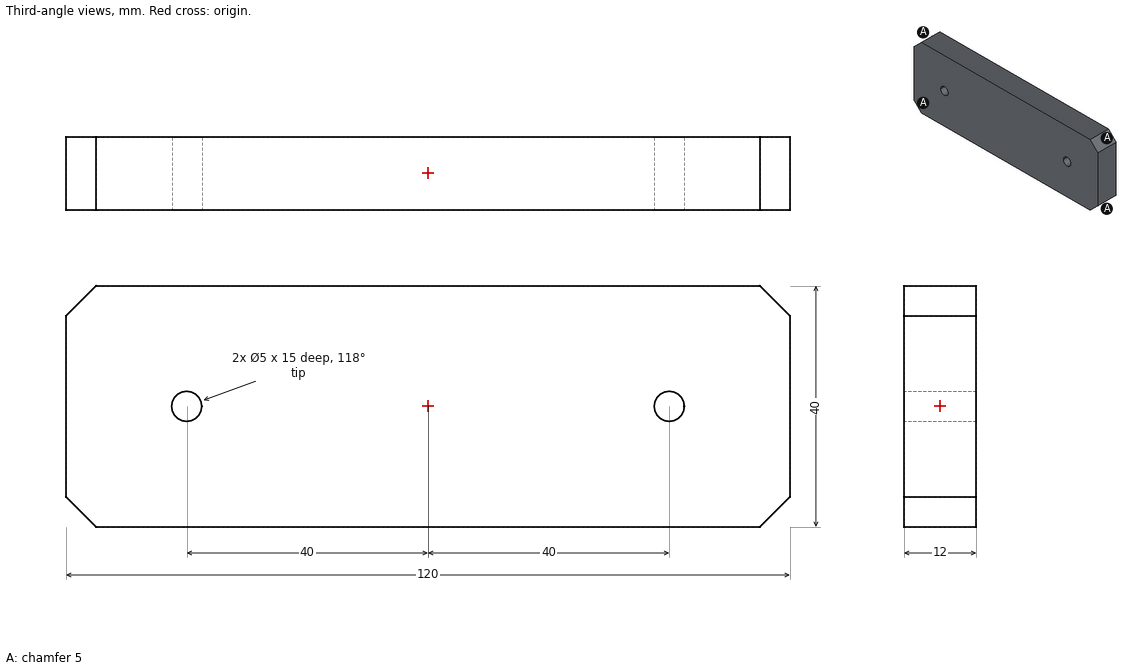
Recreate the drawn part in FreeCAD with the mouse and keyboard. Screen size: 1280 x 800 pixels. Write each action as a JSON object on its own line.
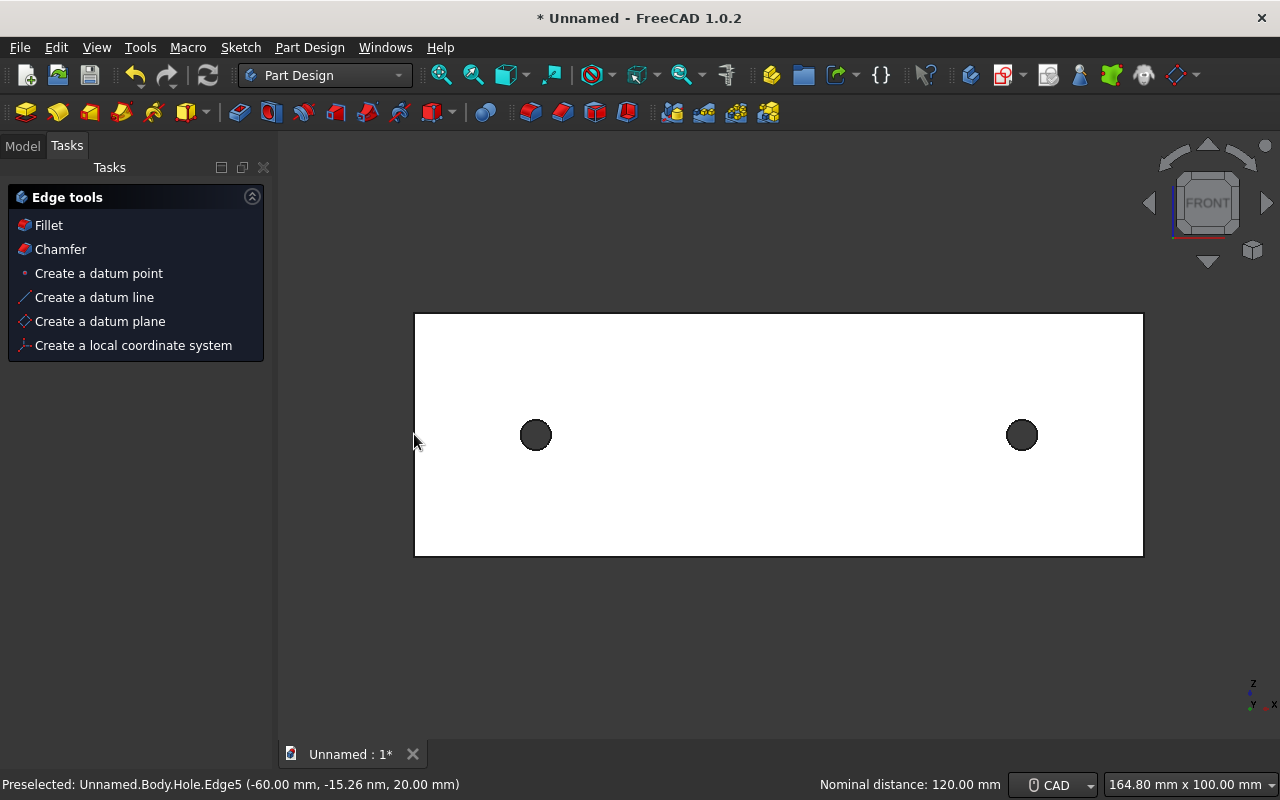
{"action": "key", "text": "3"}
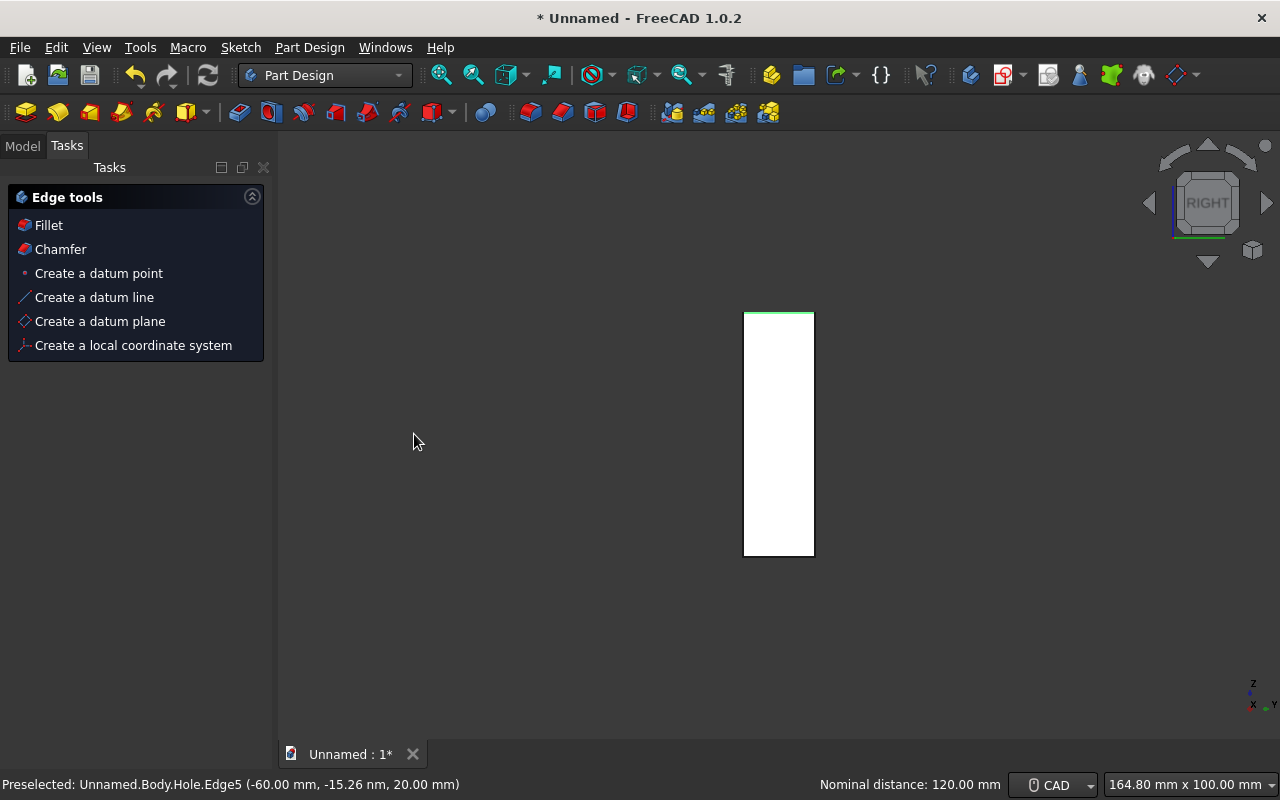
{"action": "left_click", "coordinate": [442, 76]}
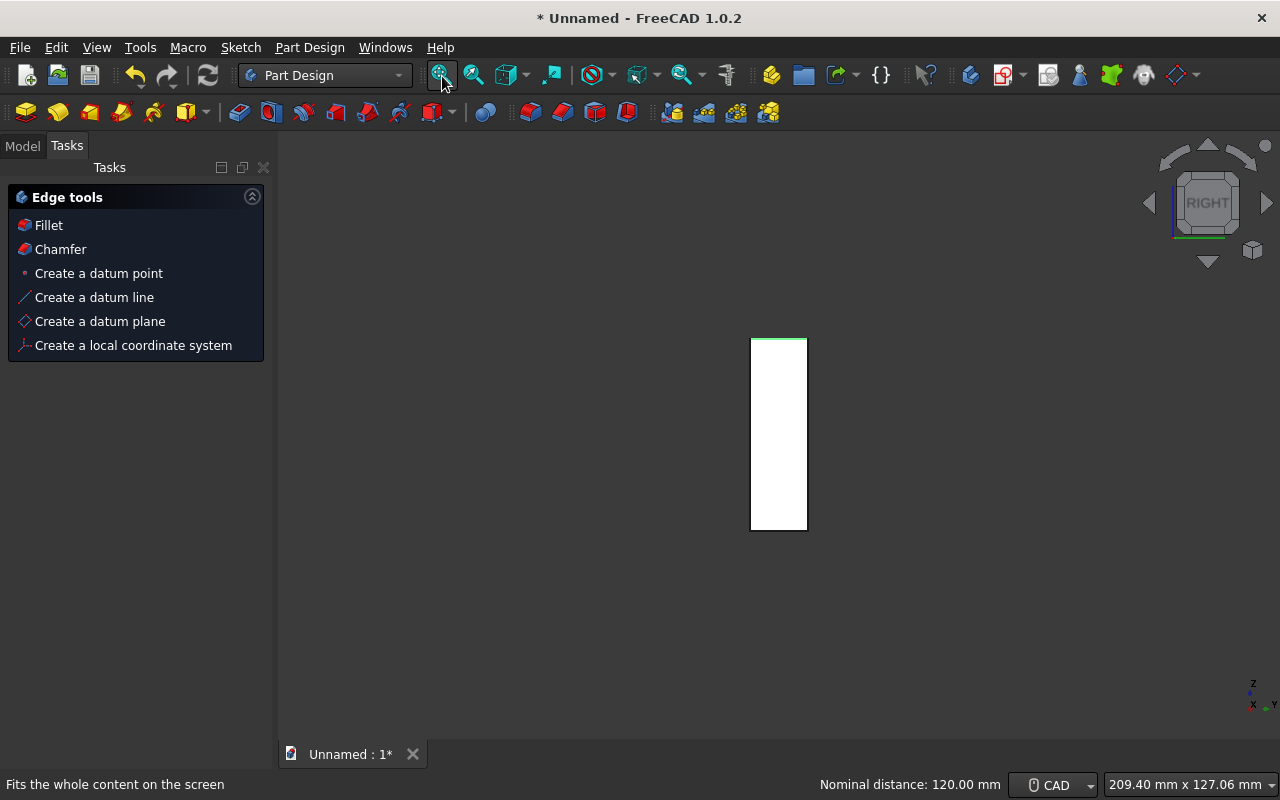
{"action": "left_click", "coordinate": [779, 530], "text": "ctrl"}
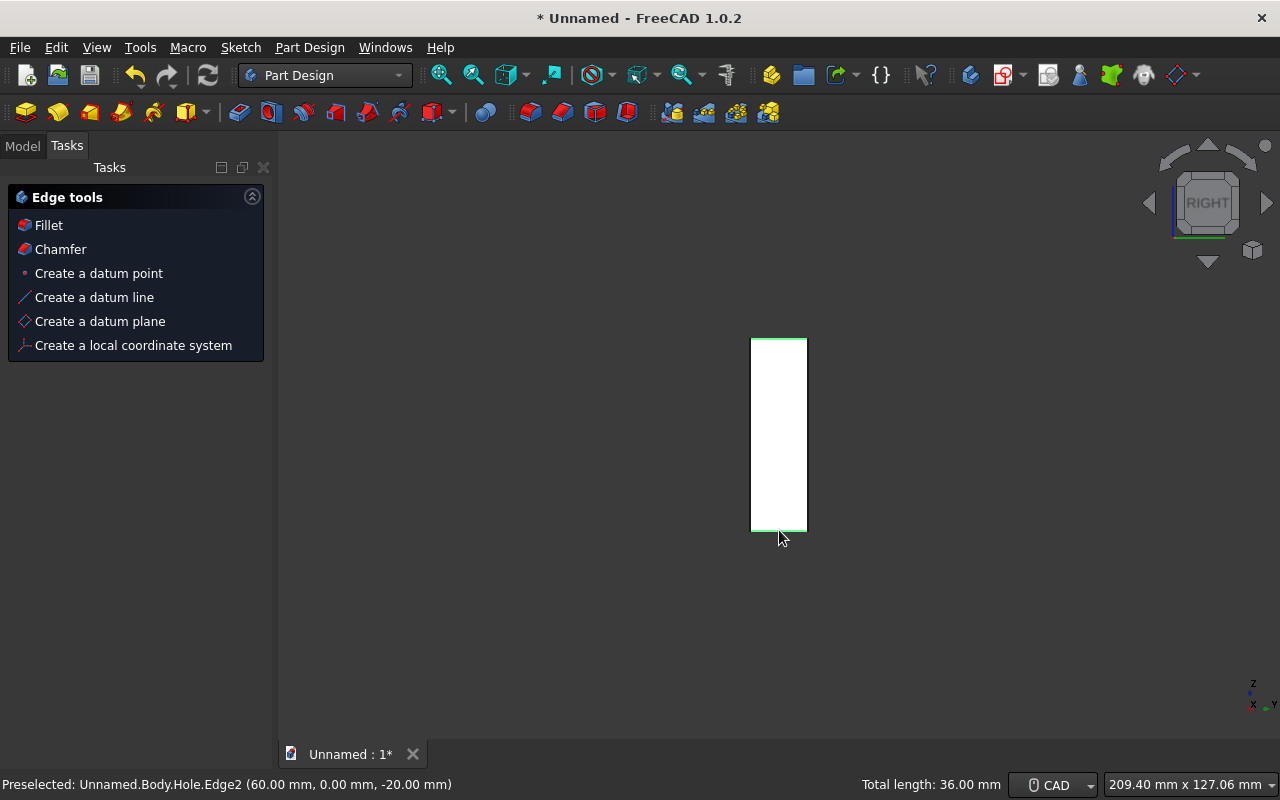
{"action": "key", "text": "5"}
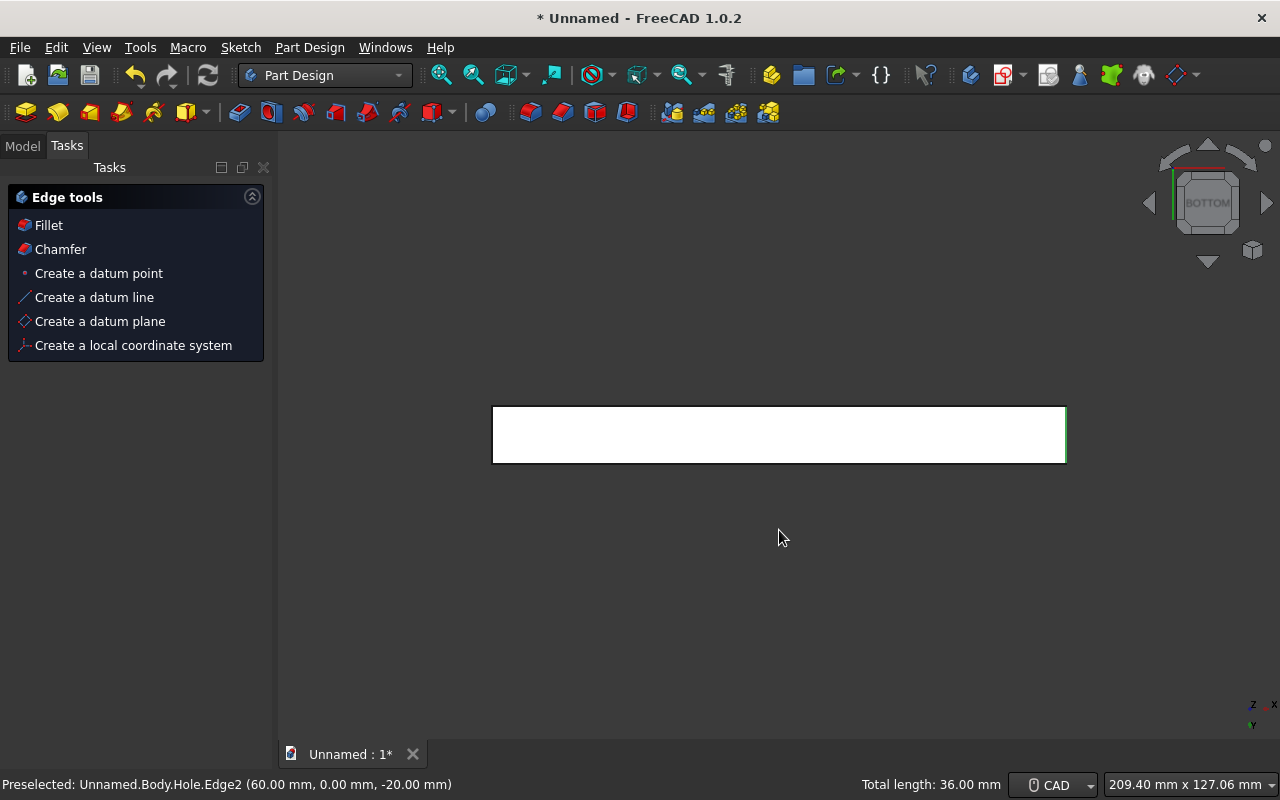
{"action": "left_click", "coordinate": [492, 434], "text": "ctrl"}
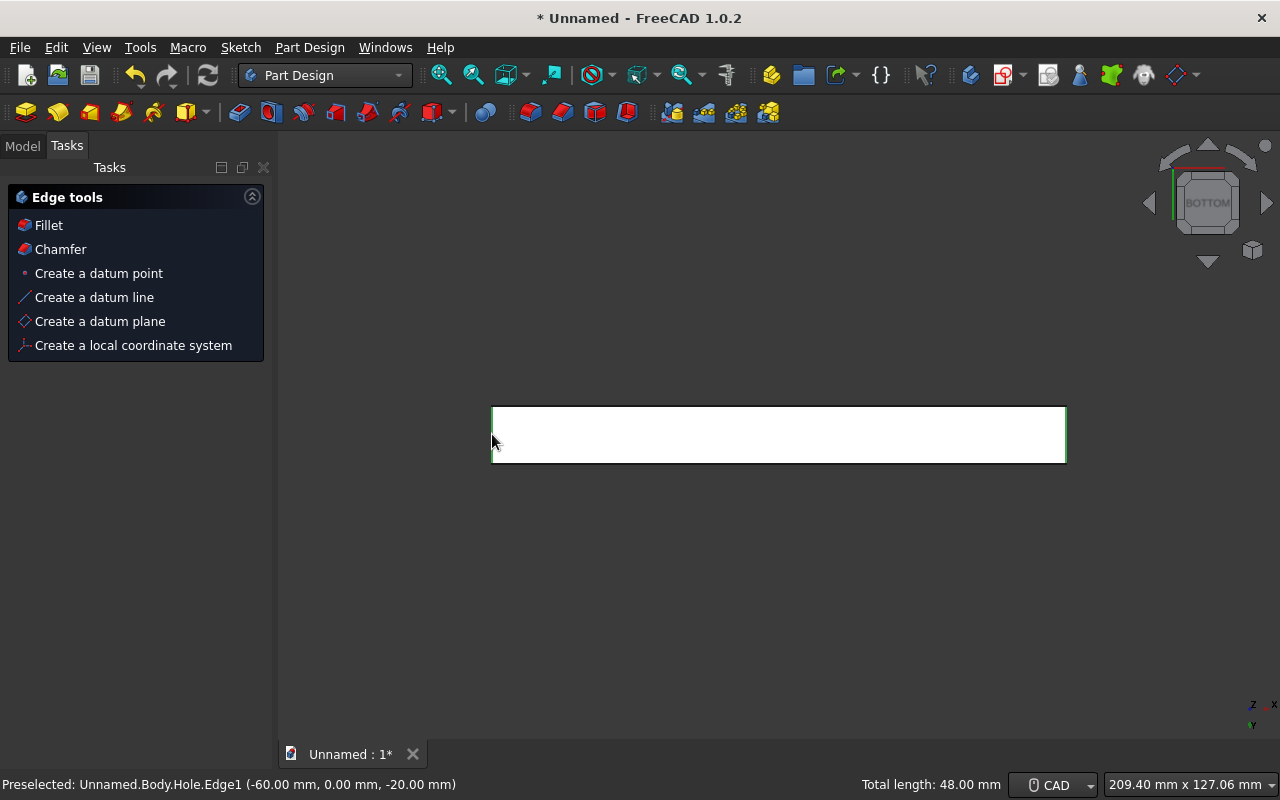
{"action": "left_click", "coordinate": [564, 112]}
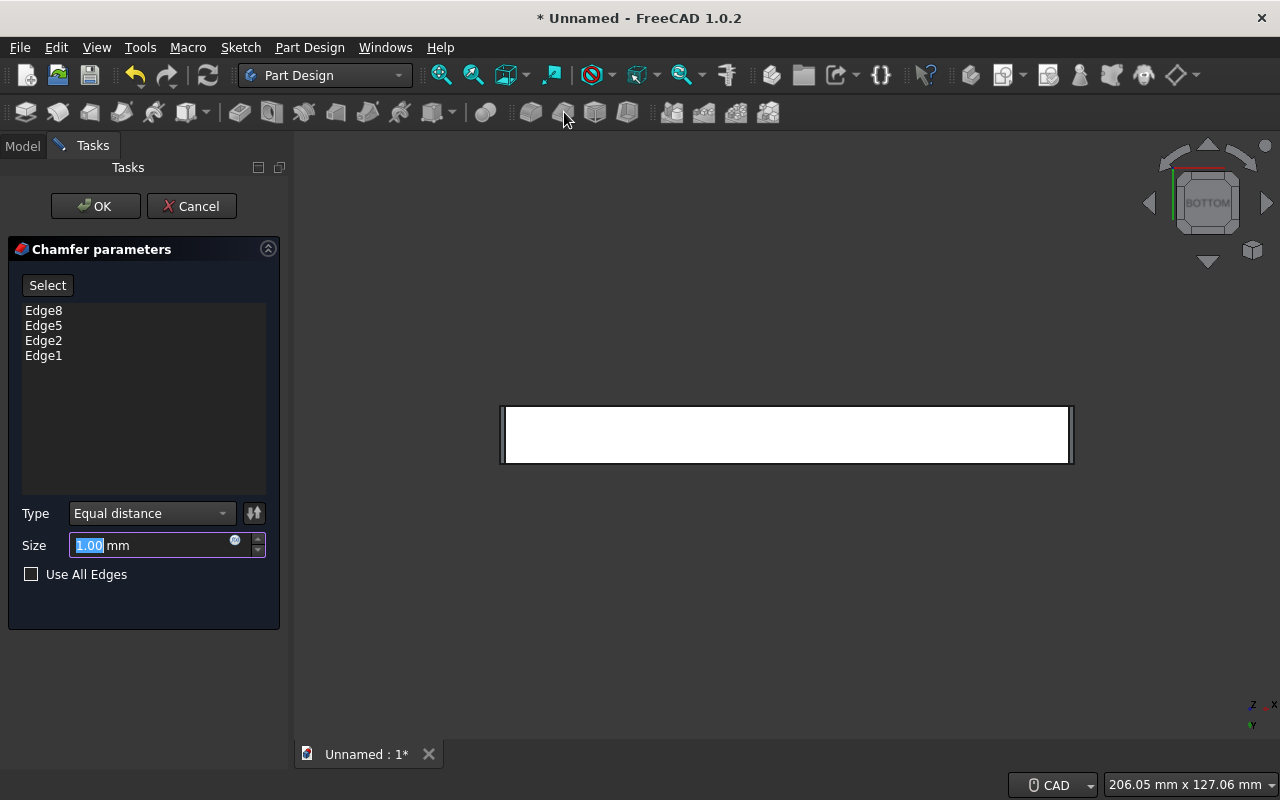
{"action": "type", "text": "5"}
{"action": "key", "text": "Tab"}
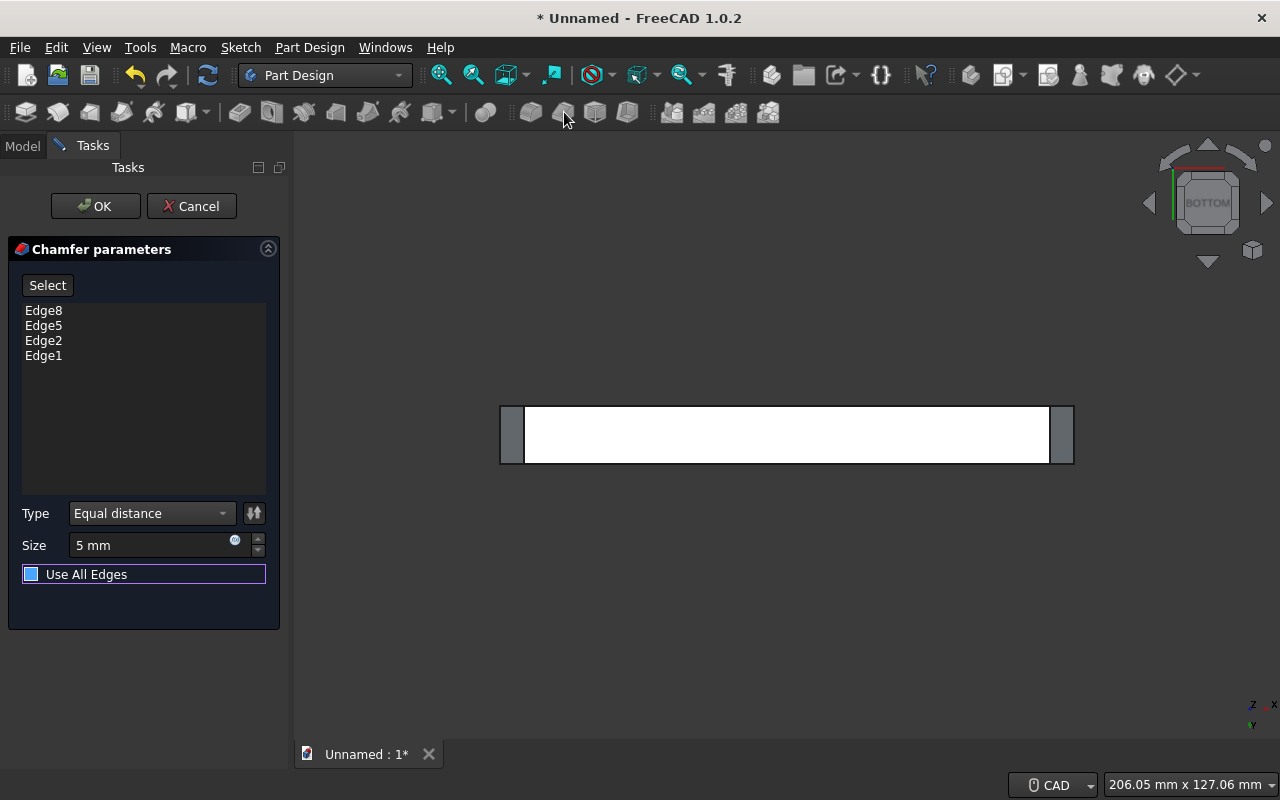
{"action": "left_click", "coordinate": [96, 206]}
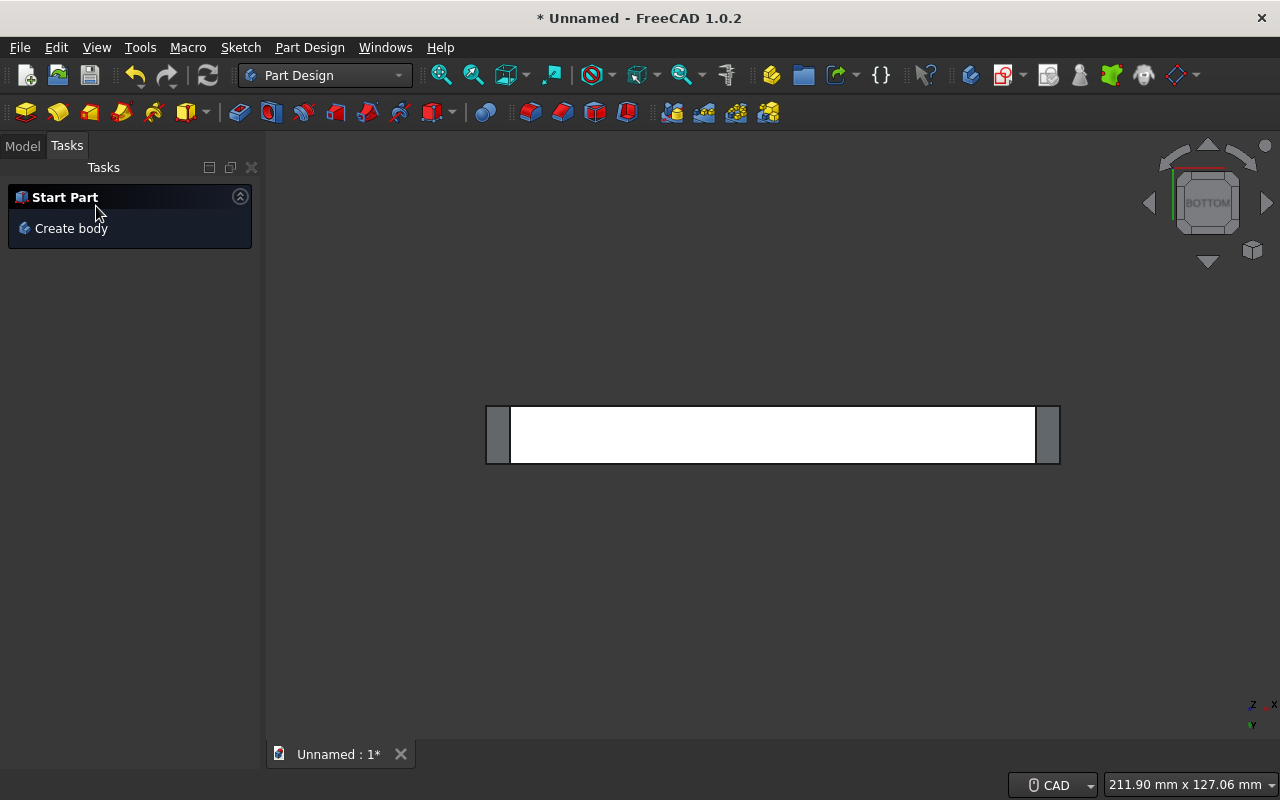
{"action": "key", "text": "0"}